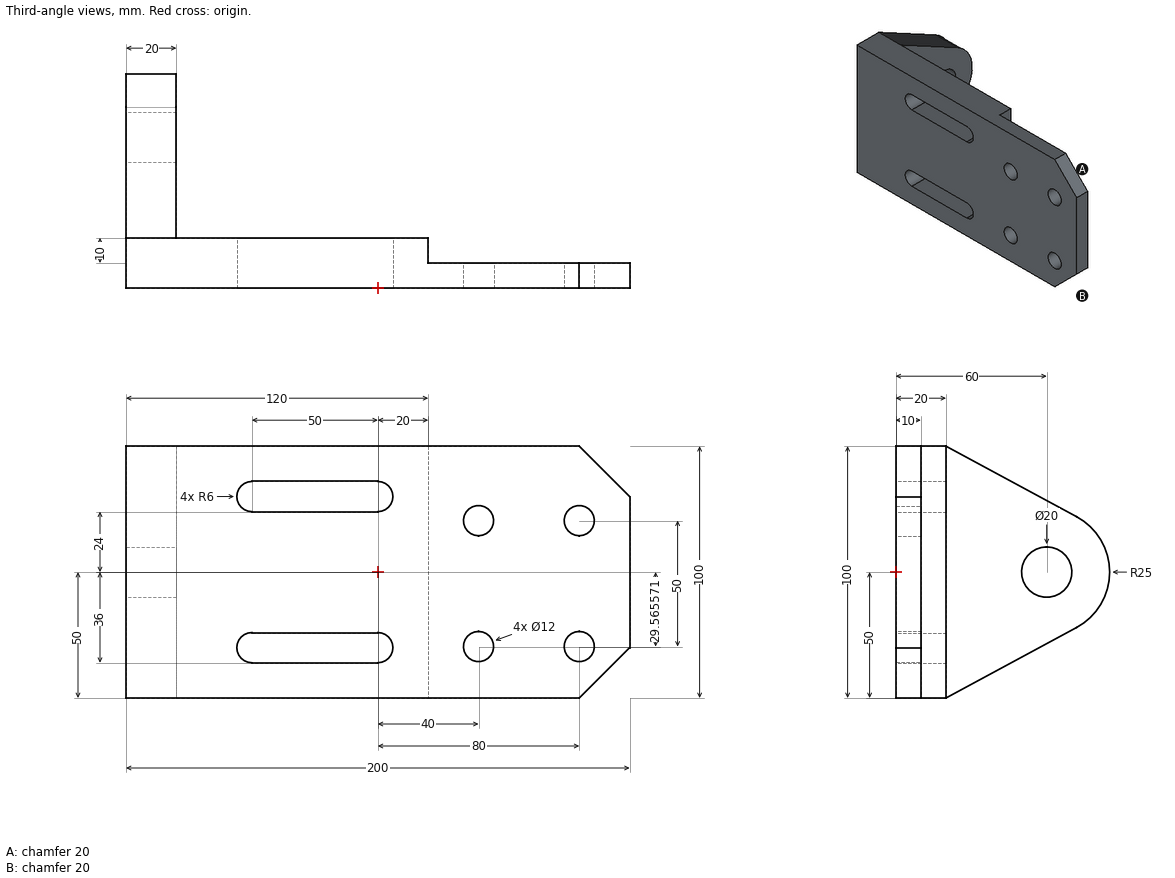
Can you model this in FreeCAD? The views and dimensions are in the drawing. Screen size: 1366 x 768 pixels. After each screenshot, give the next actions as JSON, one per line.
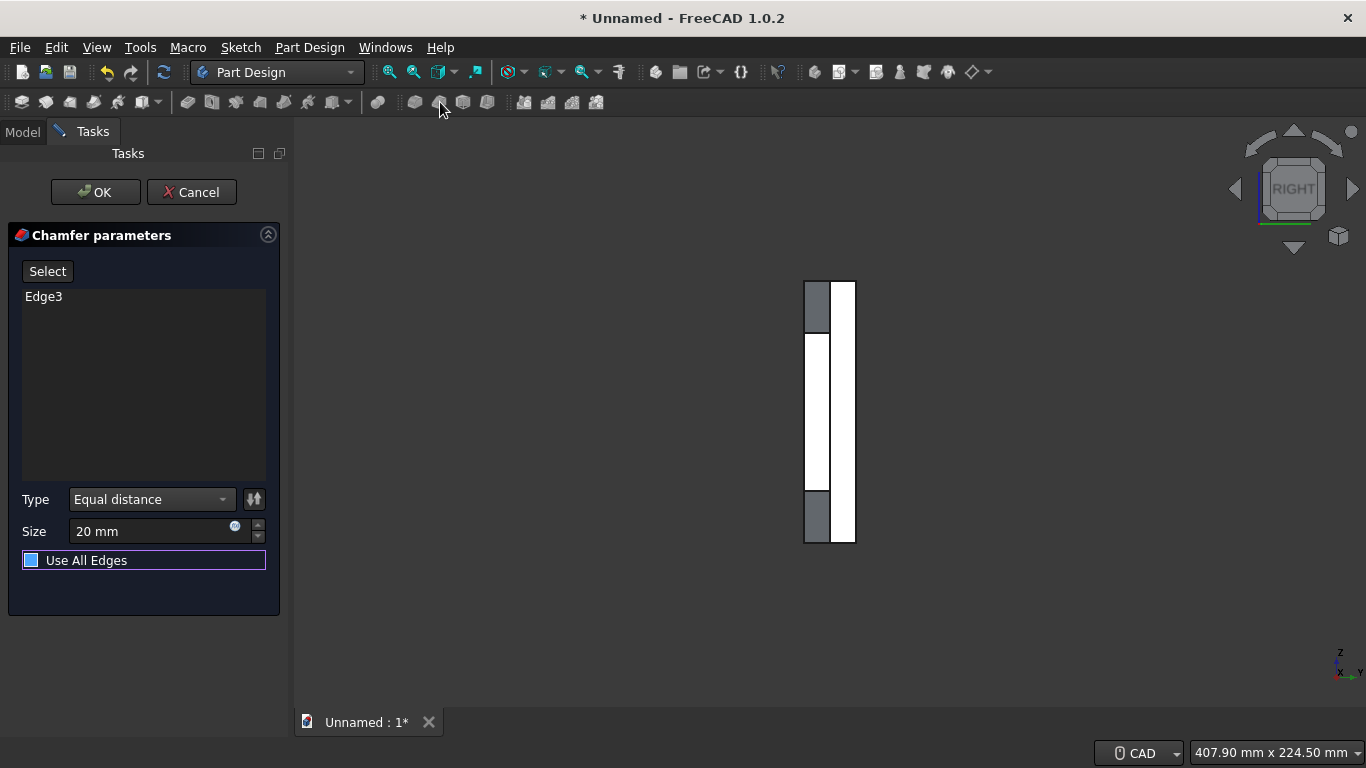
{"action": "left_click", "coordinate": [96, 192]}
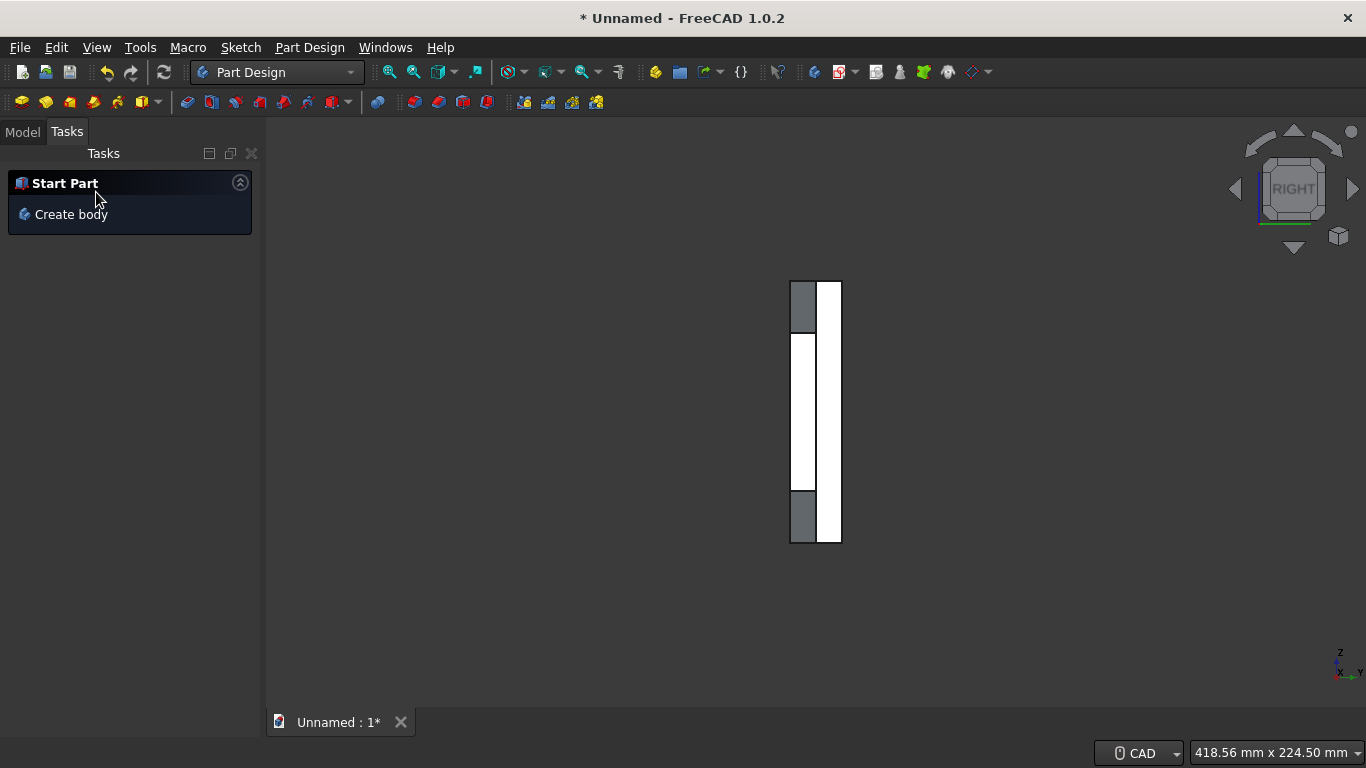
{"action": "left_click", "coordinate": [390, 72]}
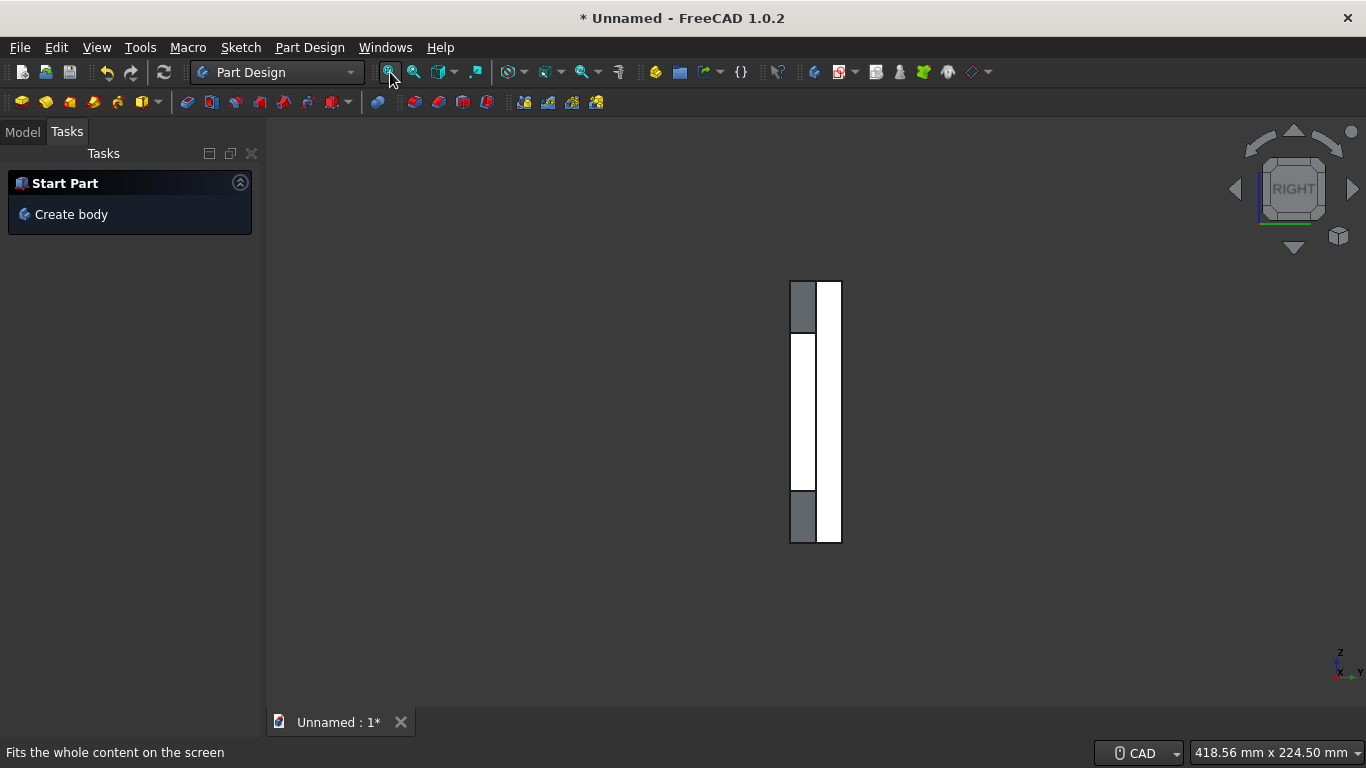
{"action": "key", "text": "4"}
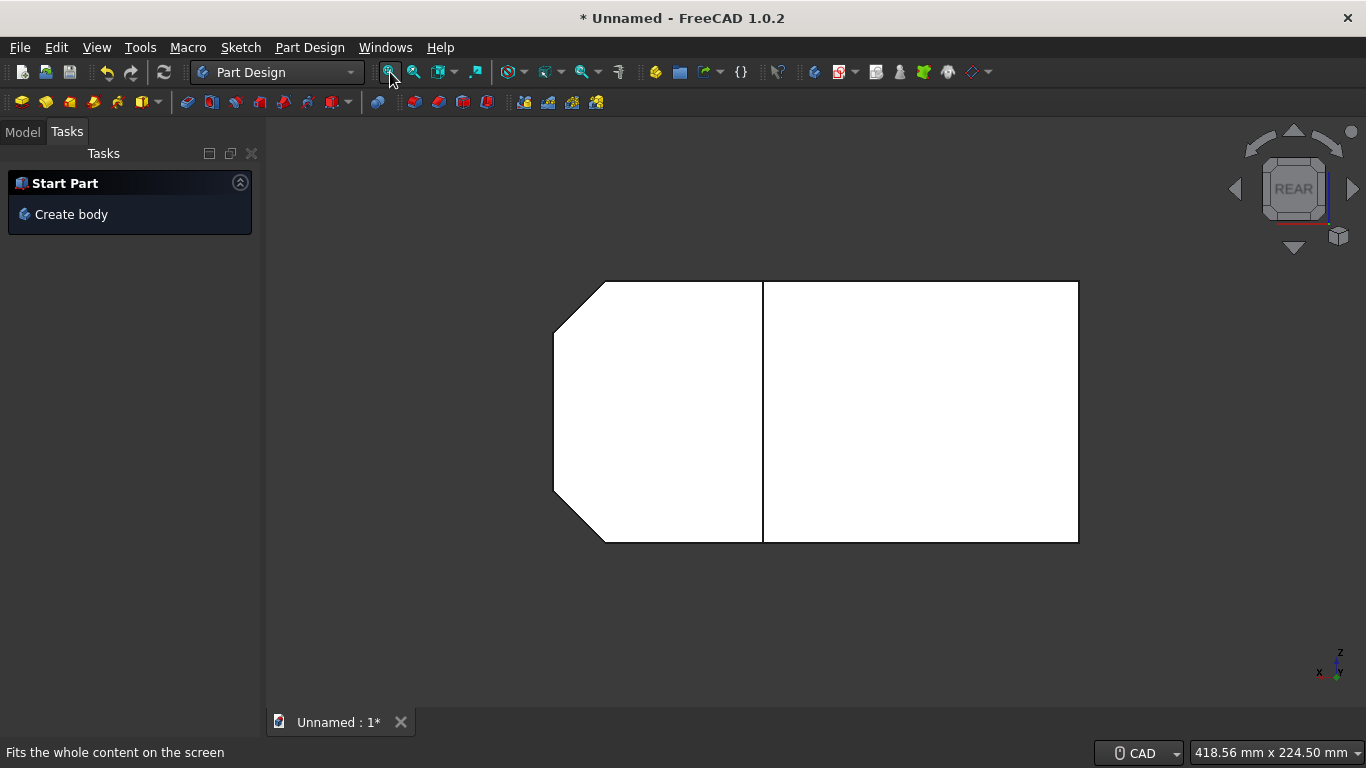
{"action": "left_click", "coordinate": [921, 411]}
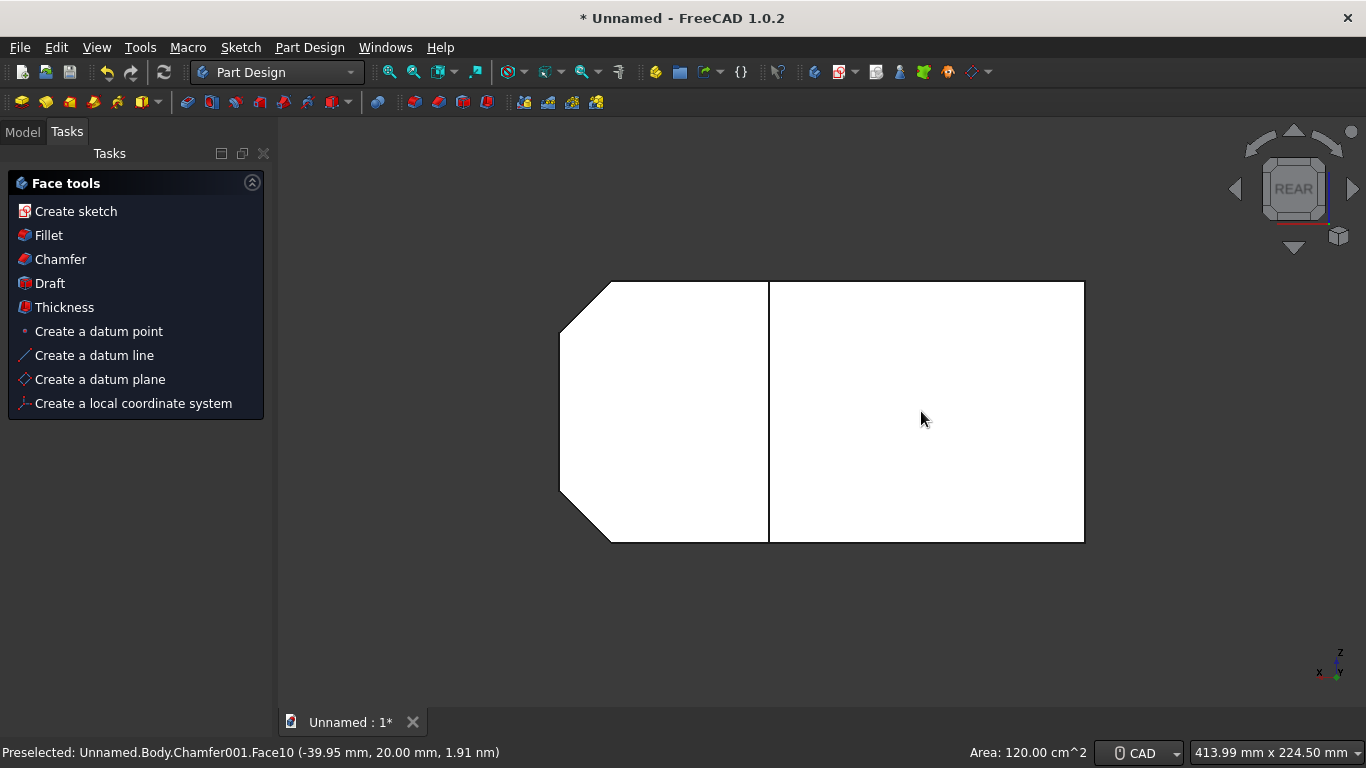
{"action": "left_click", "coordinate": [840, 72]}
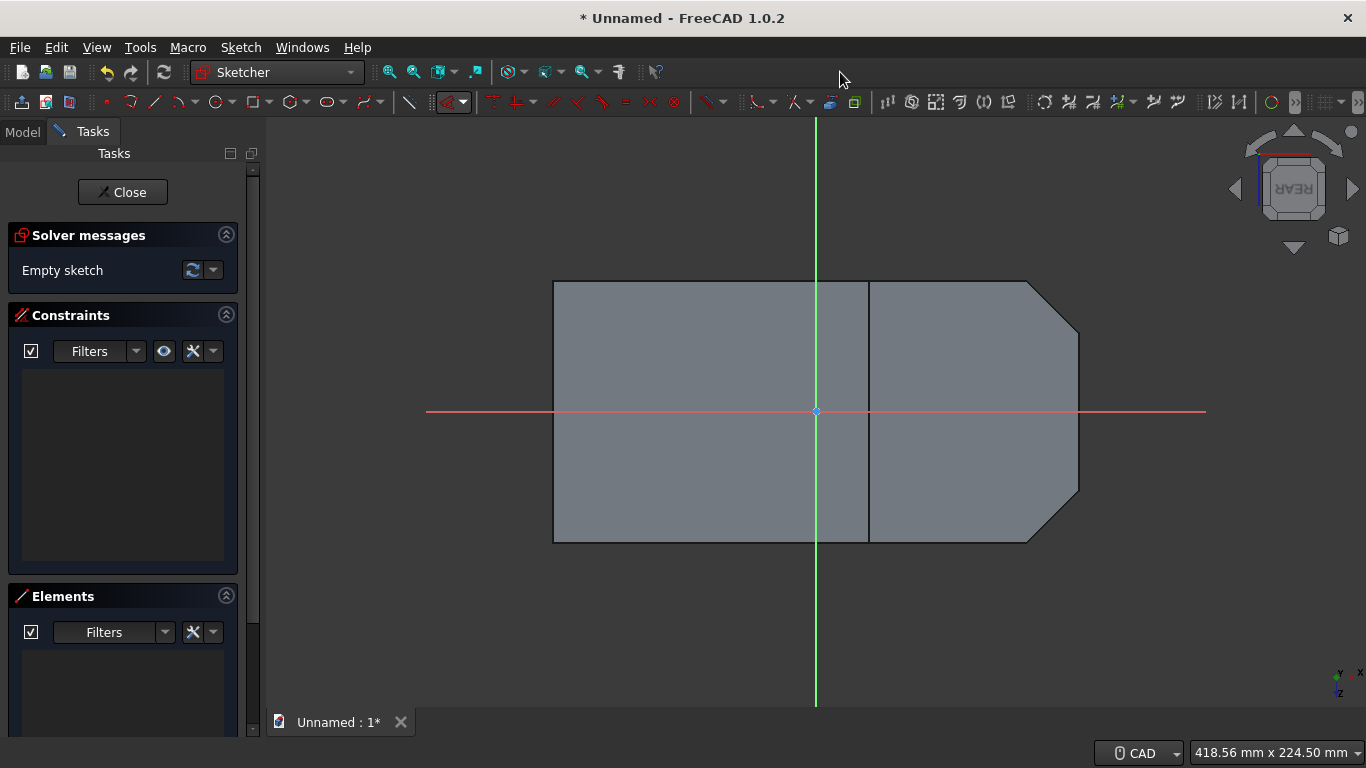
{"action": "scroll", "coordinate": [754, 412], "scroll_direction": "up", "scroll_amount": 3}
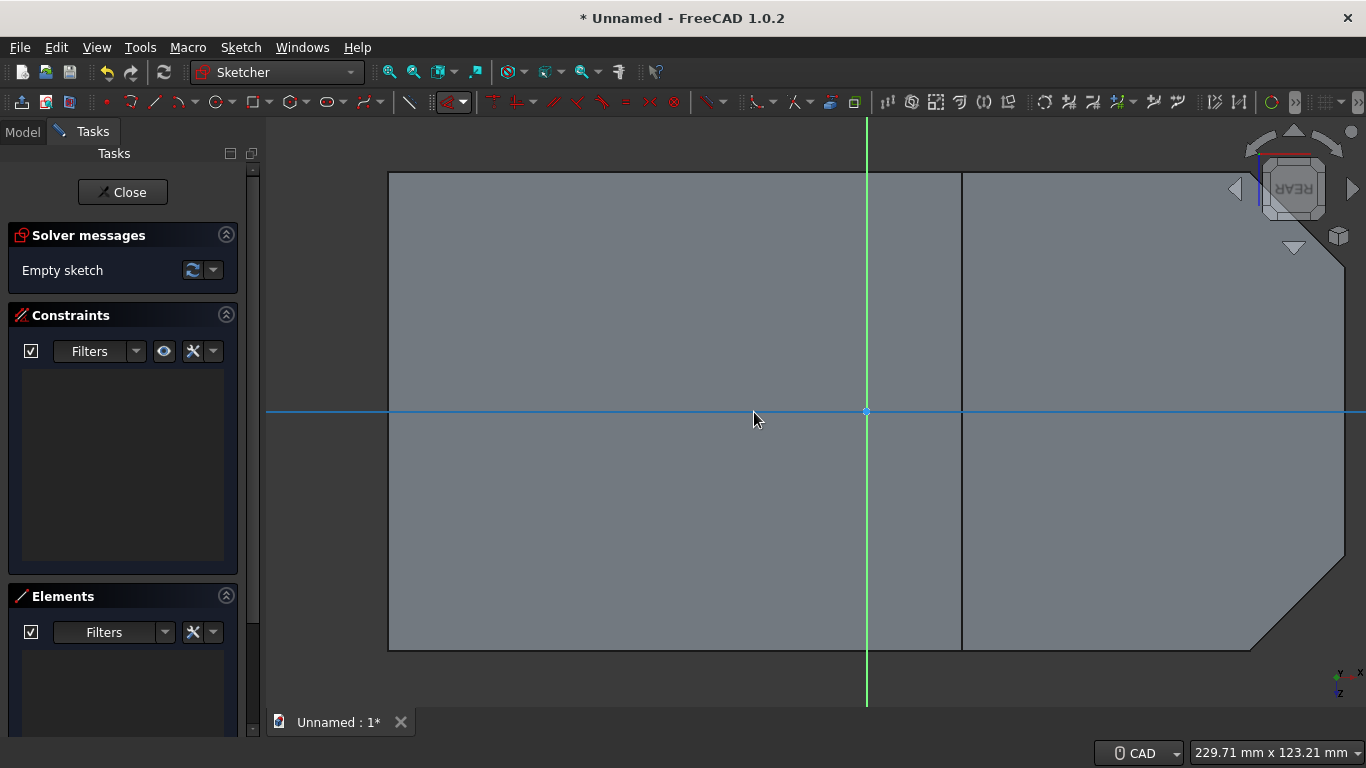
{"action": "left_click", "coordinate": [328, 102]}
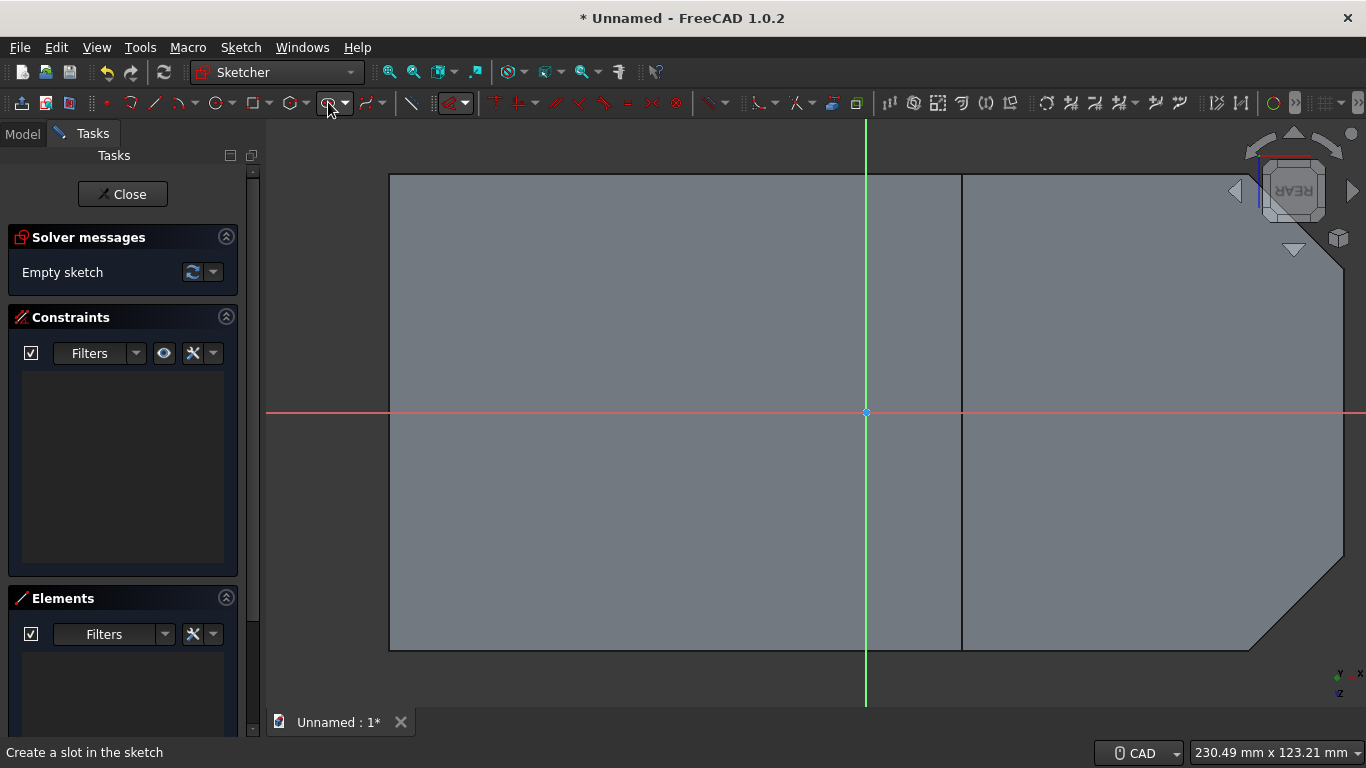
{"action": "left_click", "coordinate": [628, 556]}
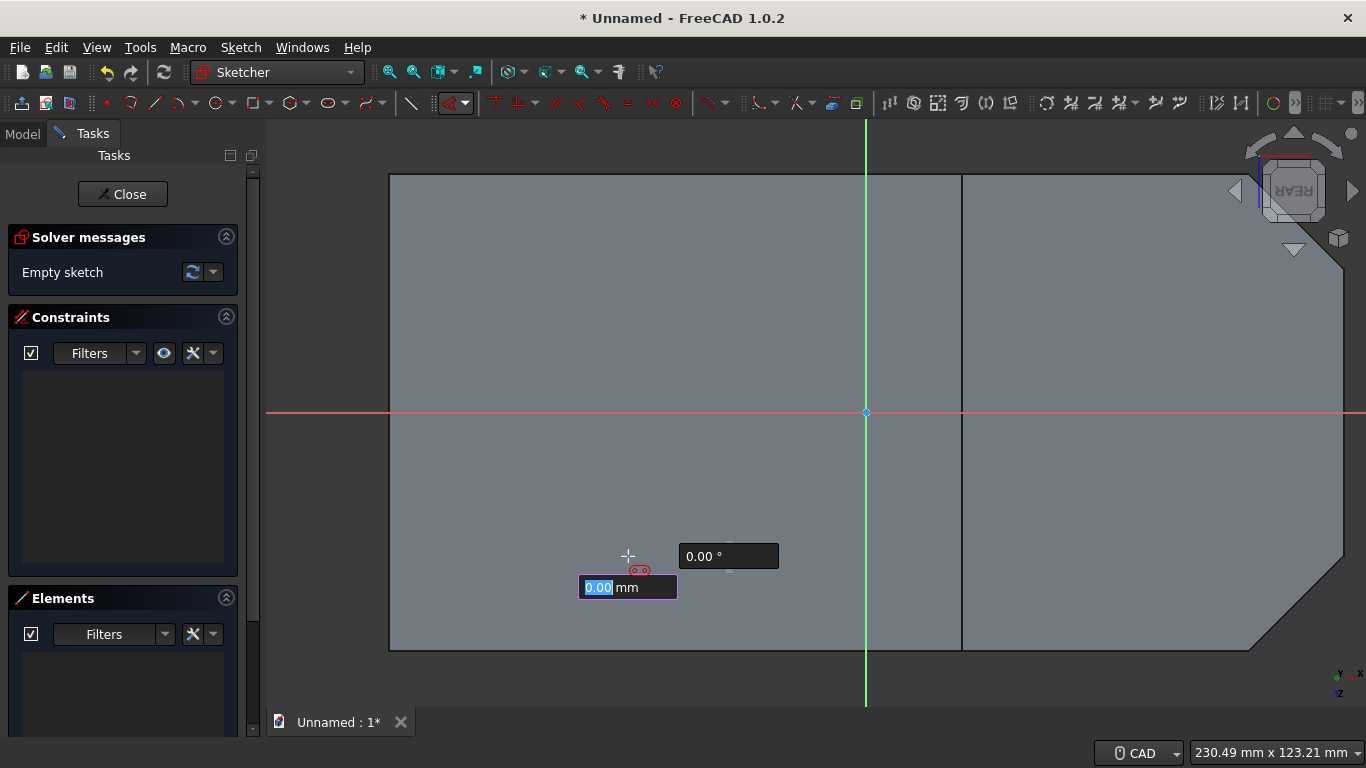
{"action": "left_click", "coordinate": [866, 556]}